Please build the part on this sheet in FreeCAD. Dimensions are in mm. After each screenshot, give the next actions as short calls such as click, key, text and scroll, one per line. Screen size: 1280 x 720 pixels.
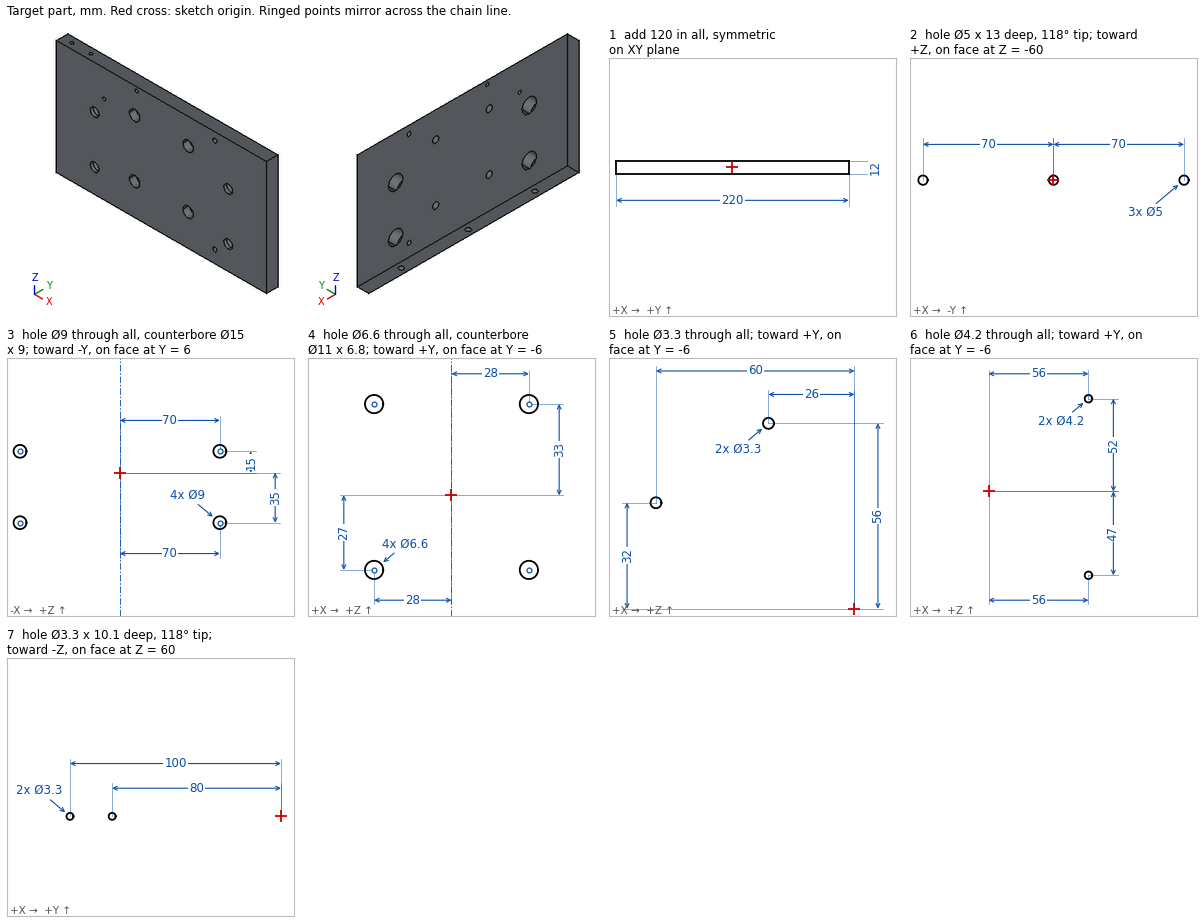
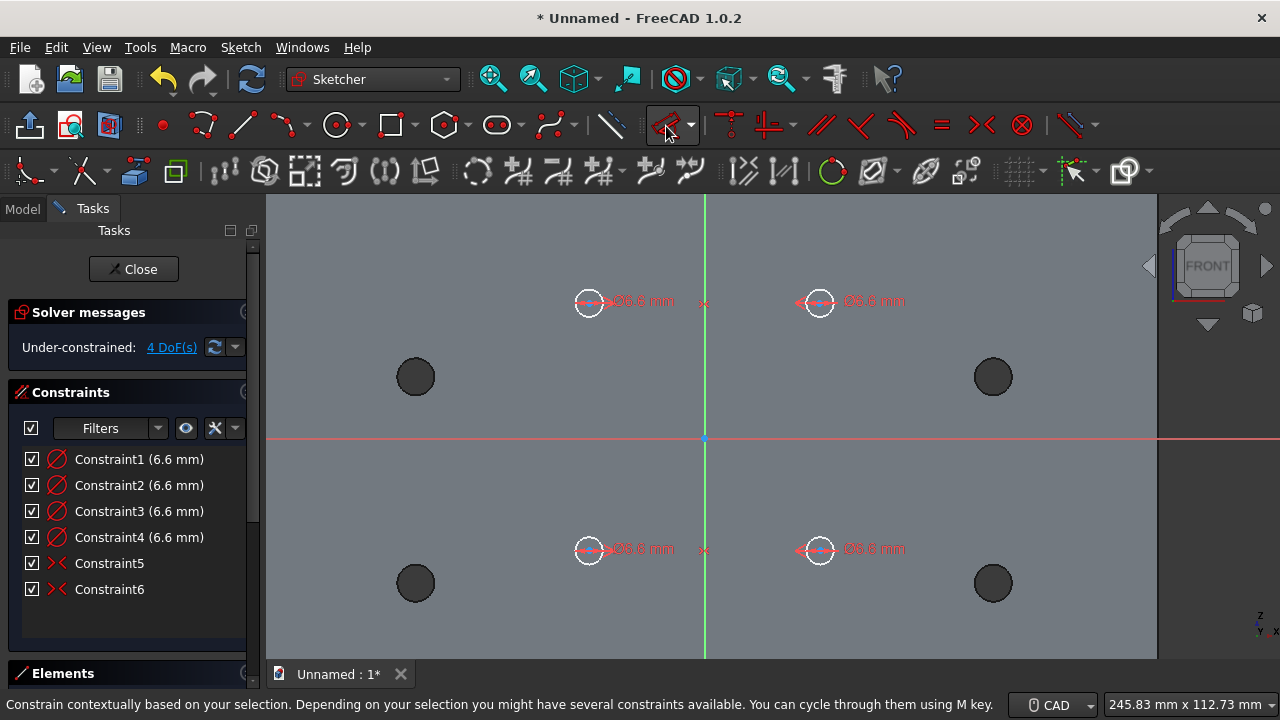
click(589, 551)
click(647, 585)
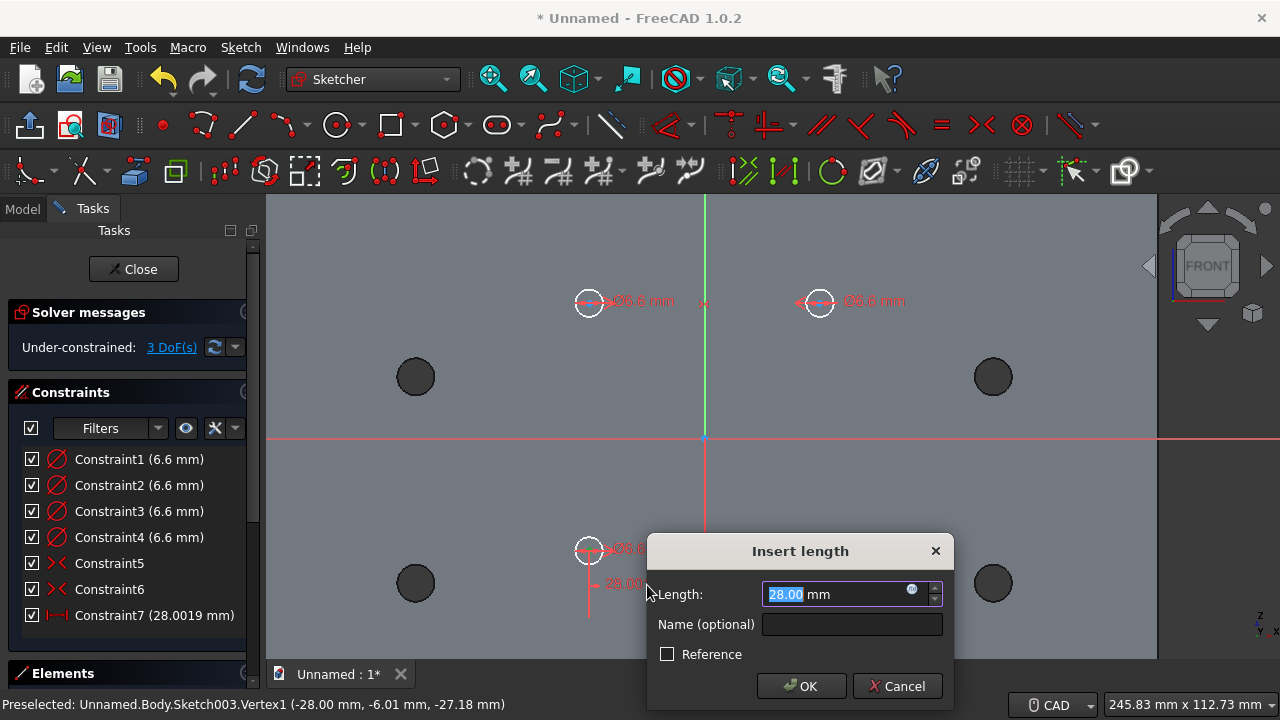
text(28)
key(Return)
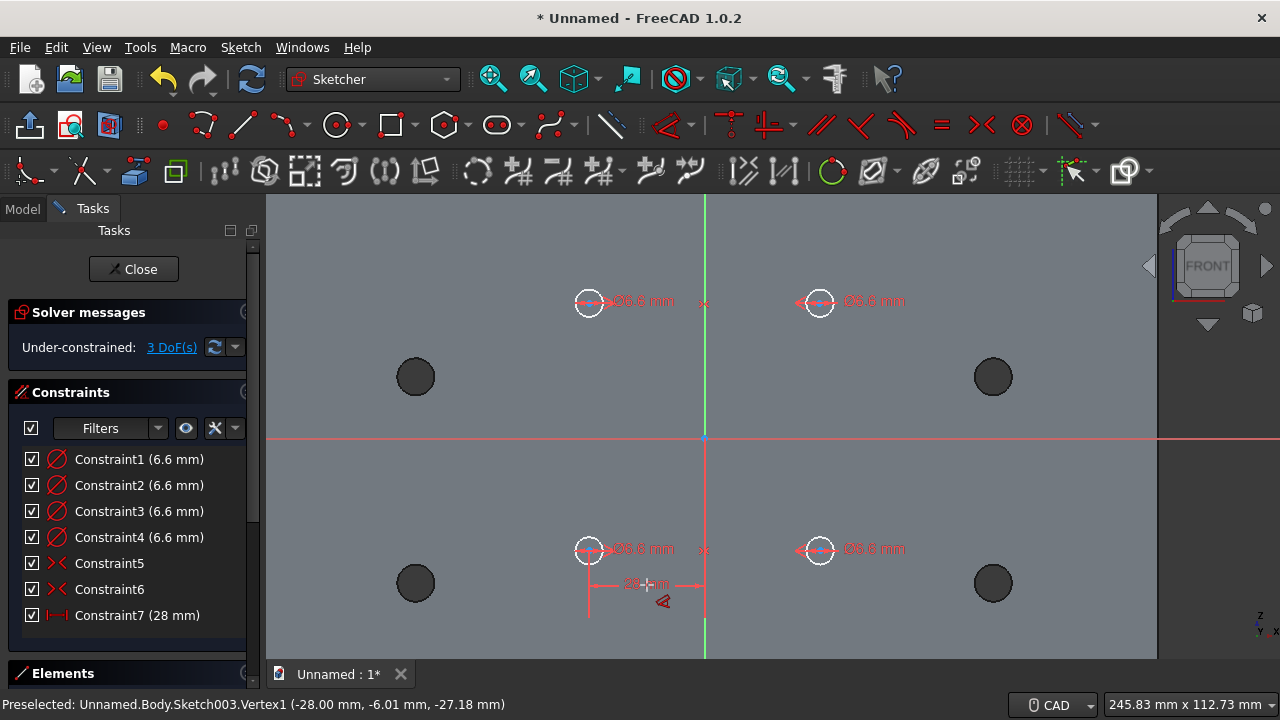
click(589, 551)
click(555, 495)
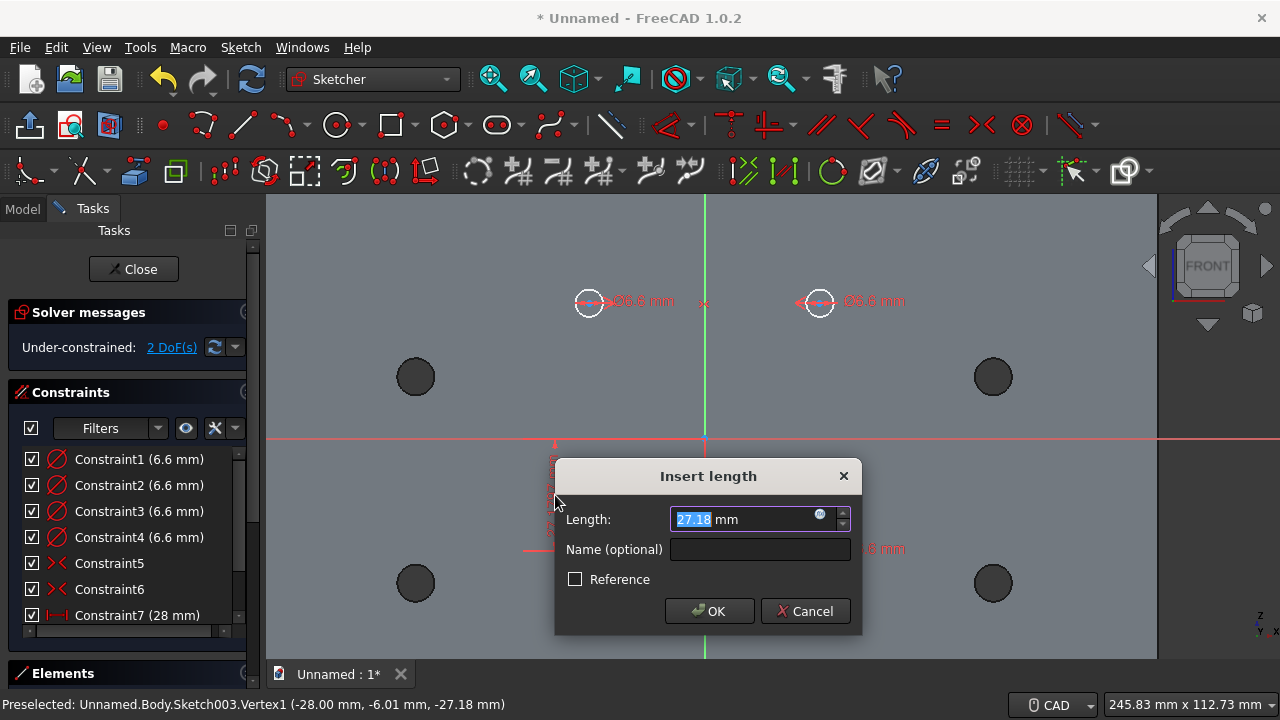
text(27)
key(Return)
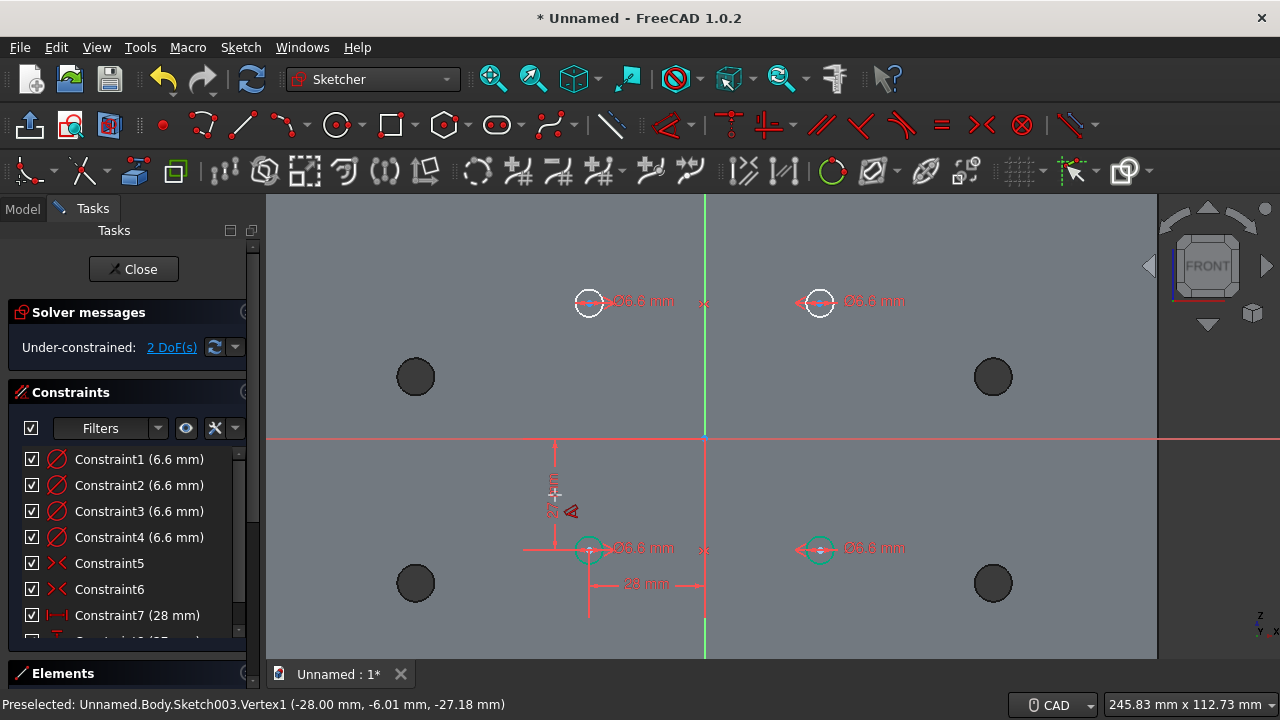
click(820, 303)
click(762, 269)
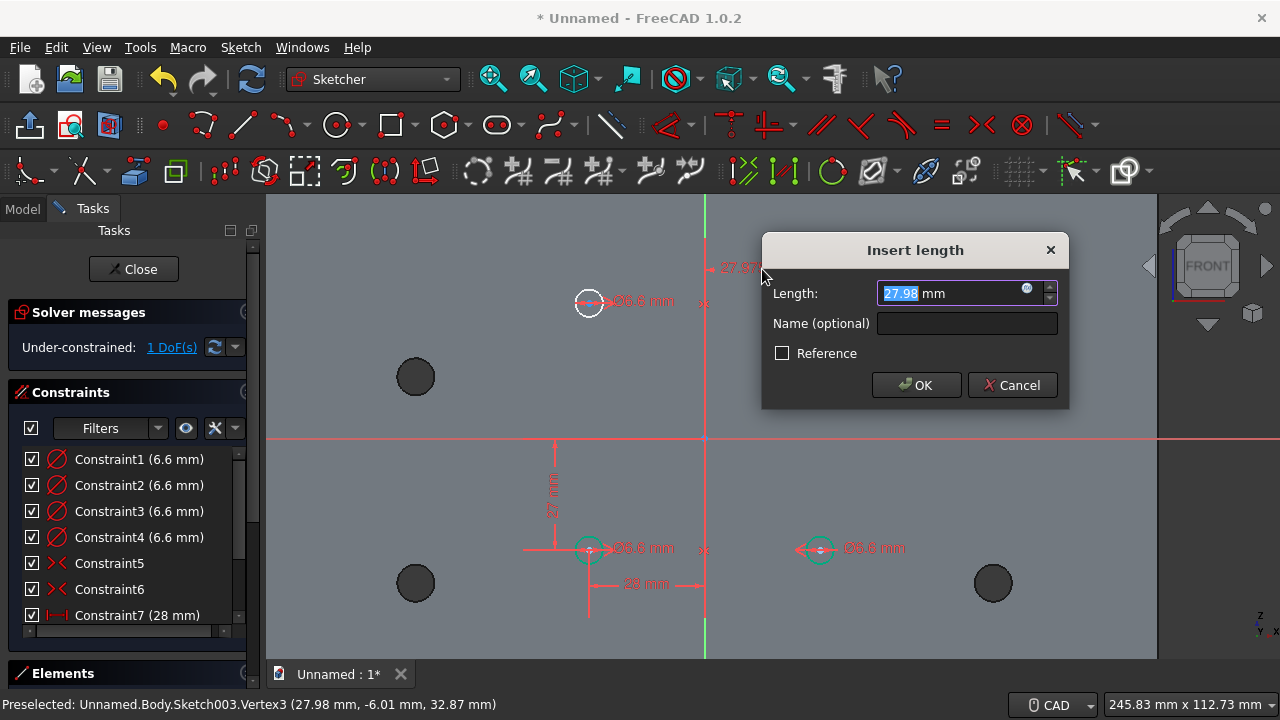
text(28)
key(Return)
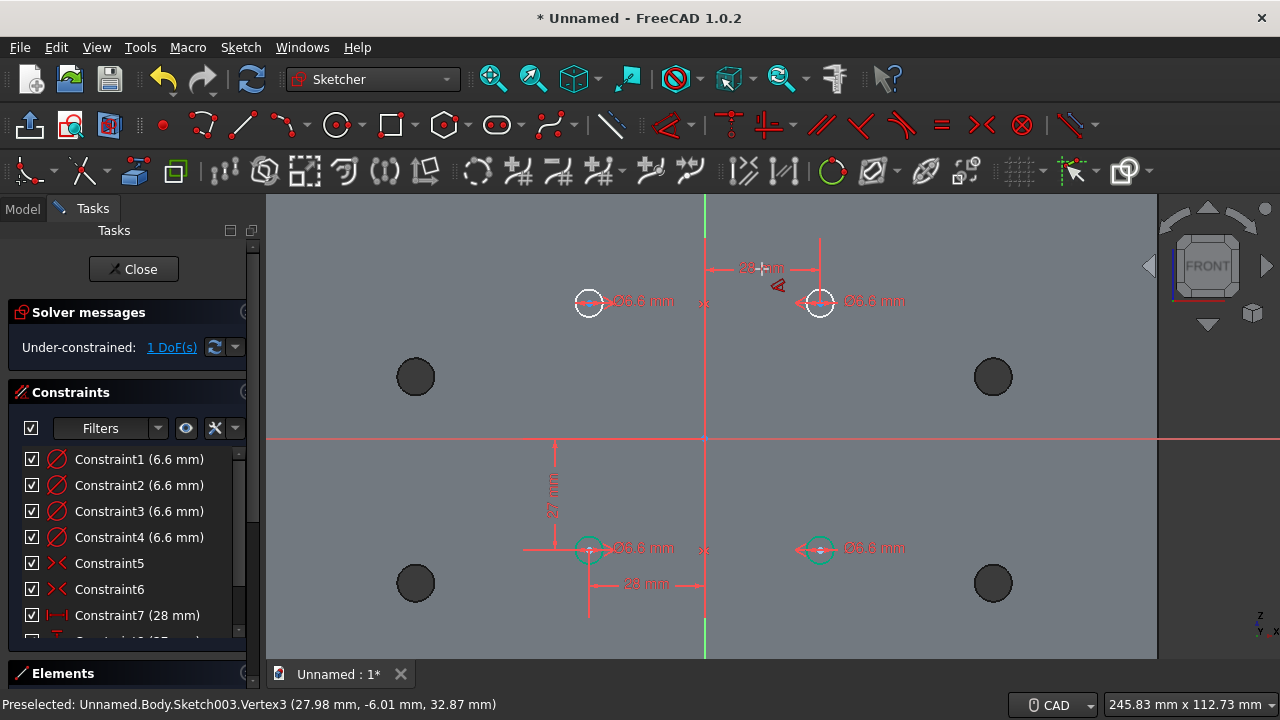
click(820, 303)
click(854, 371)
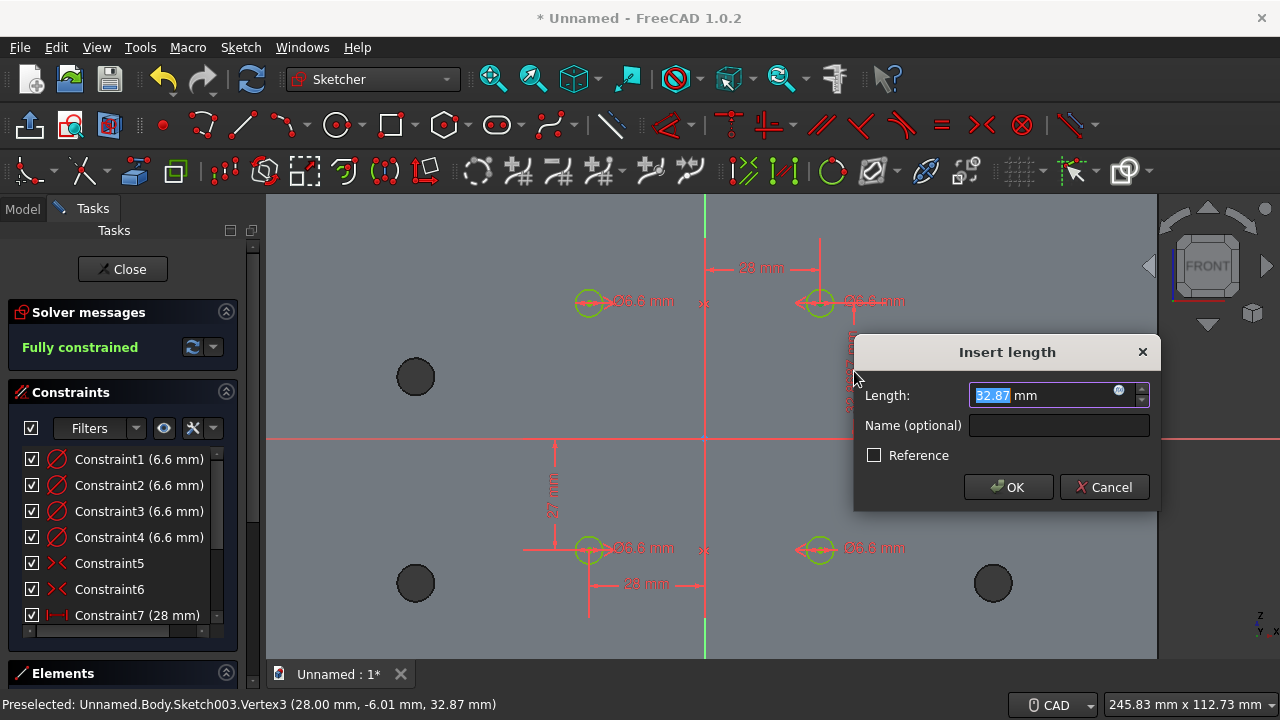
text(33)
key(Return)
key(Escape)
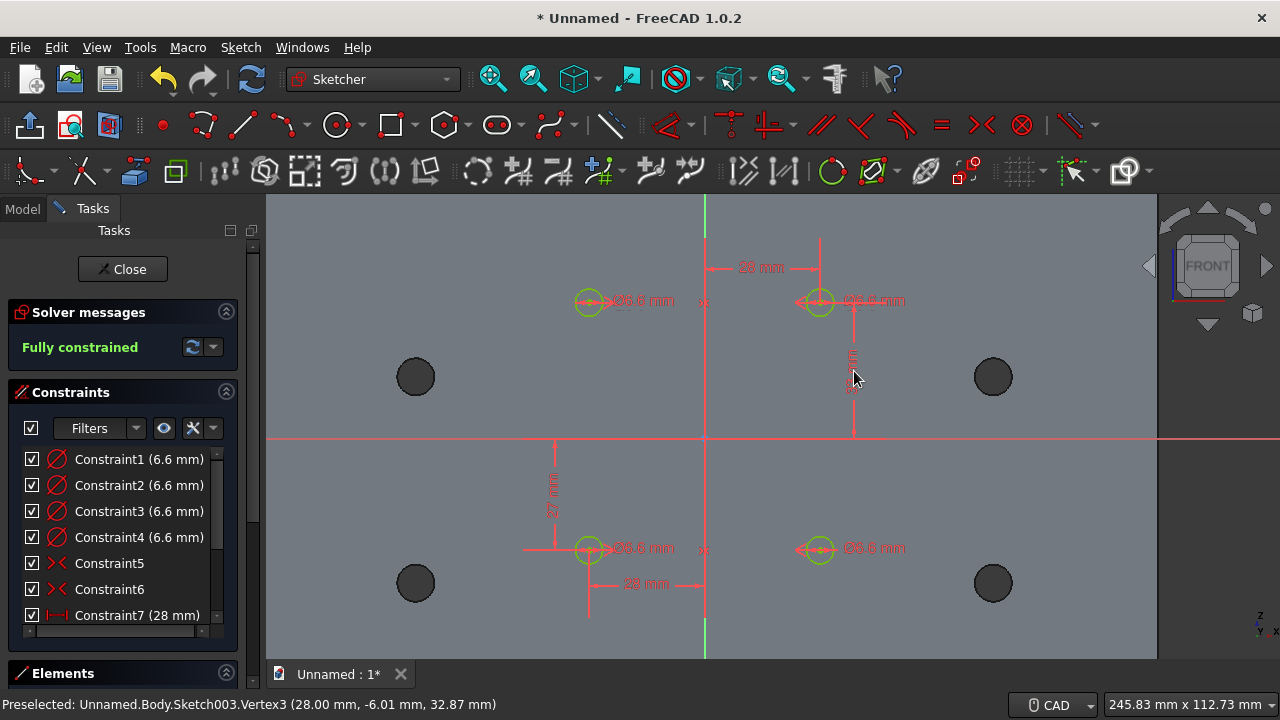
click(123, 269)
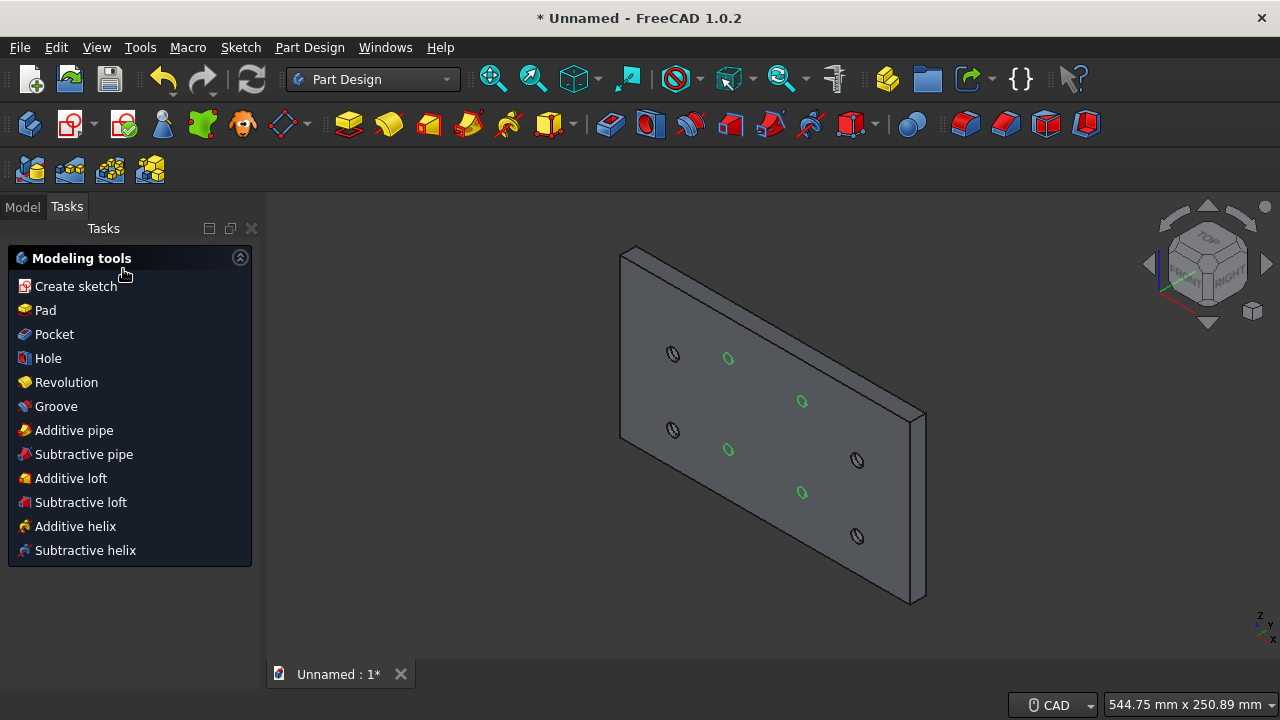
click(652, 124)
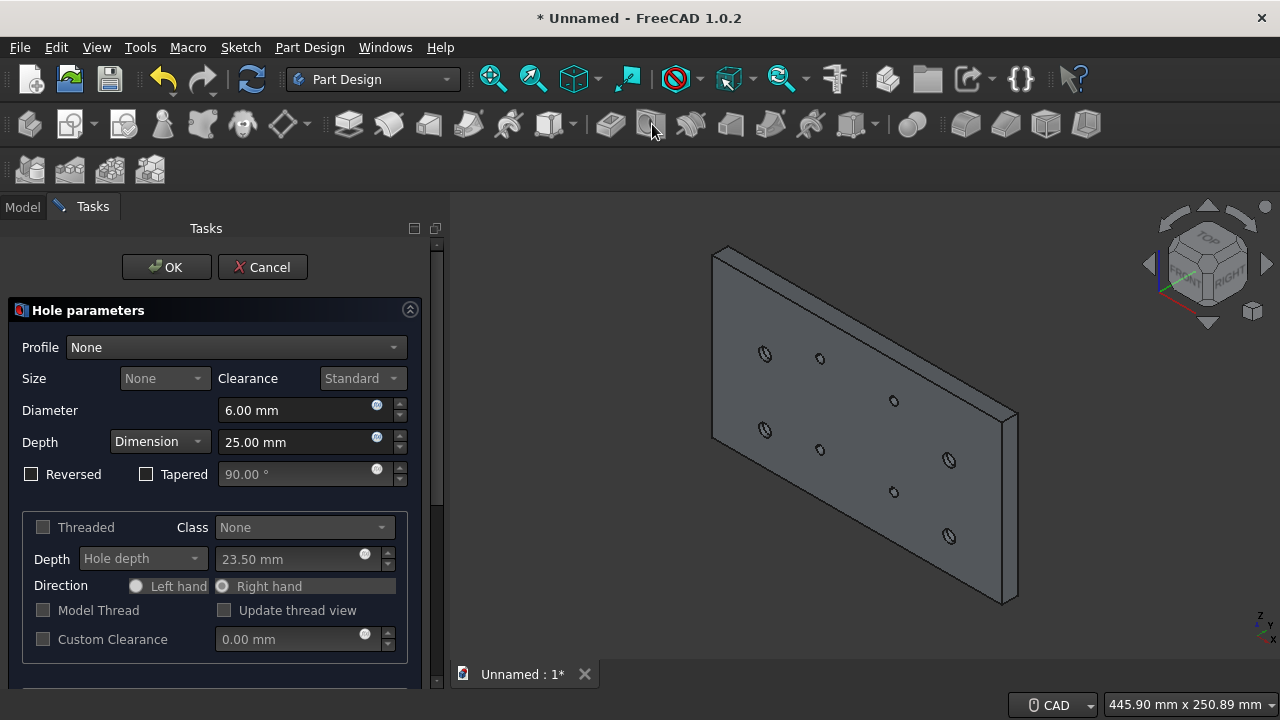
triple_click(305, 410)